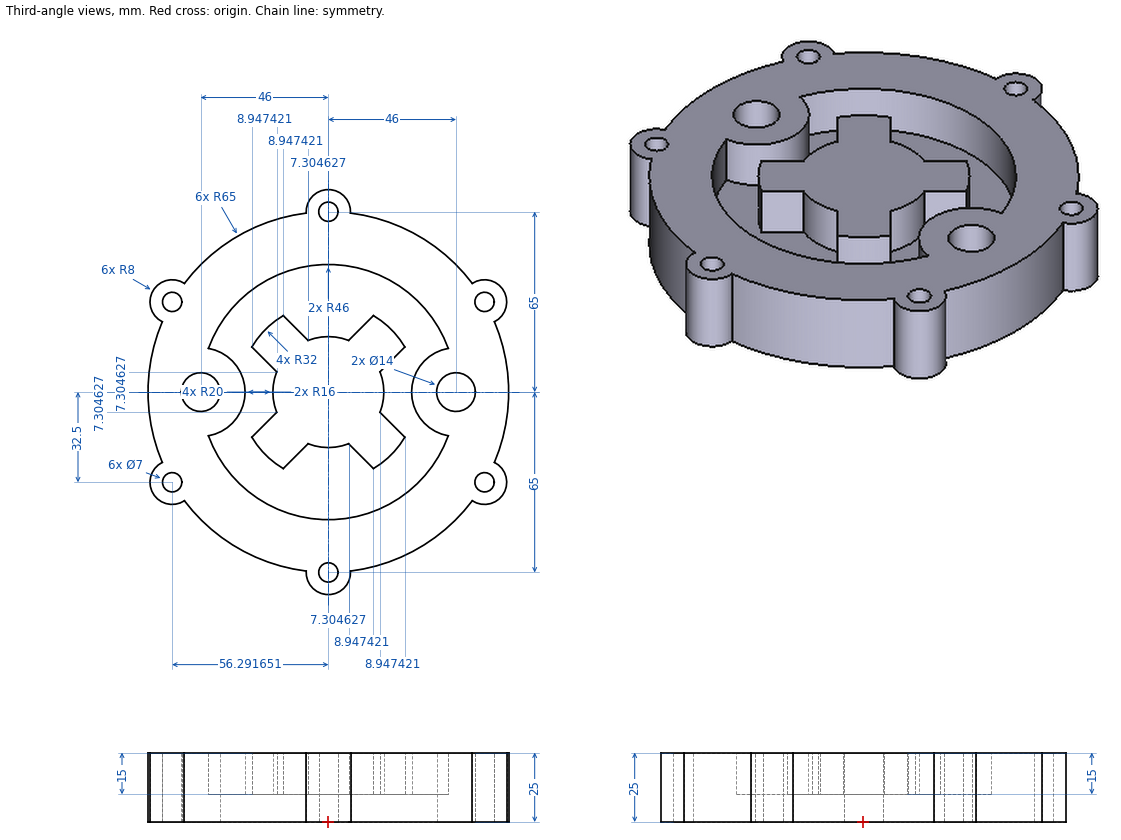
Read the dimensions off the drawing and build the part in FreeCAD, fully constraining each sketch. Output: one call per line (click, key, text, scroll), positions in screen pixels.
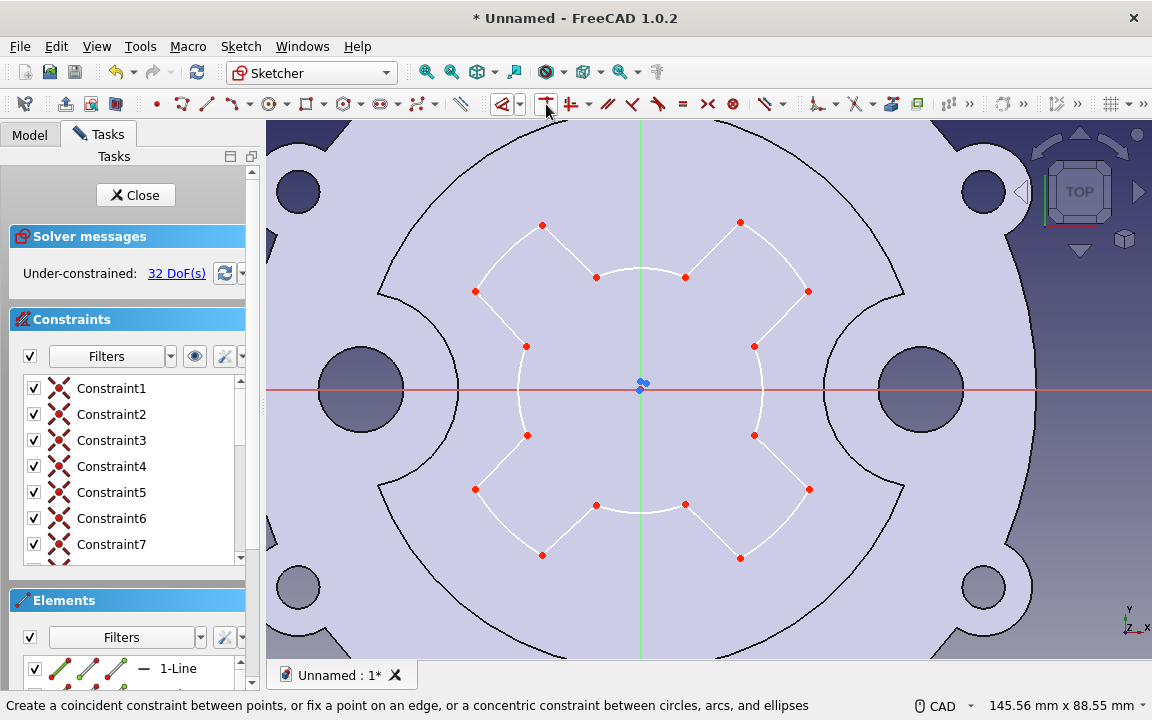
click(519, 241)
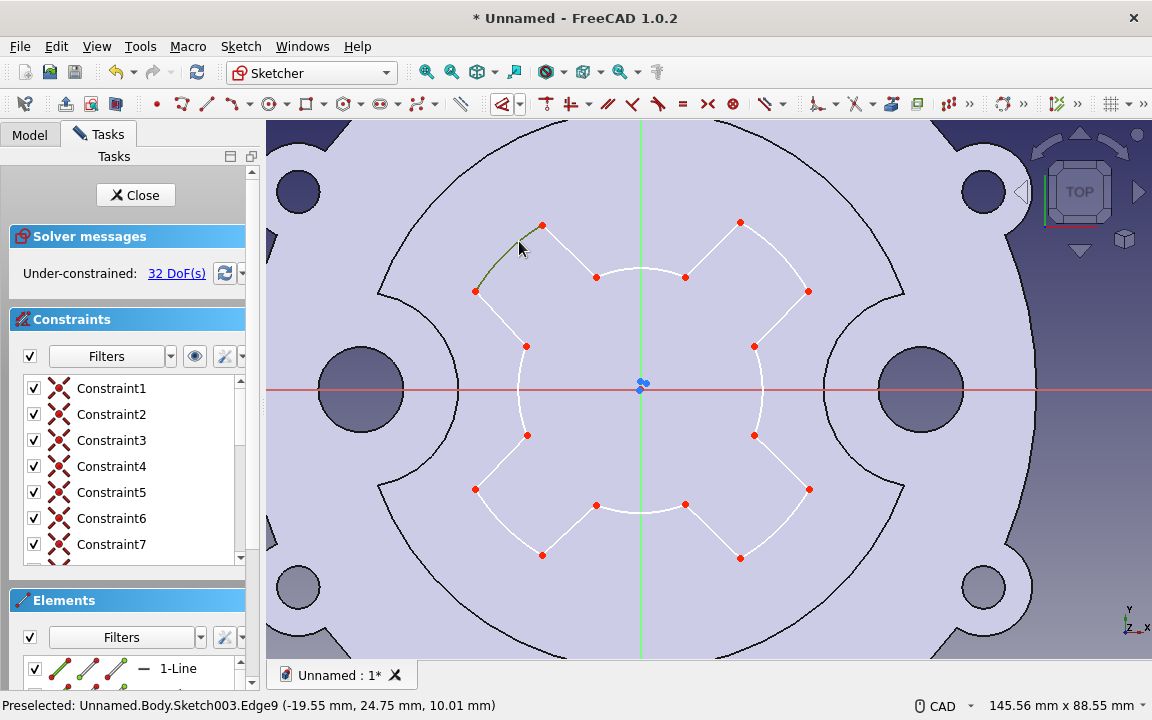
click(761, 409)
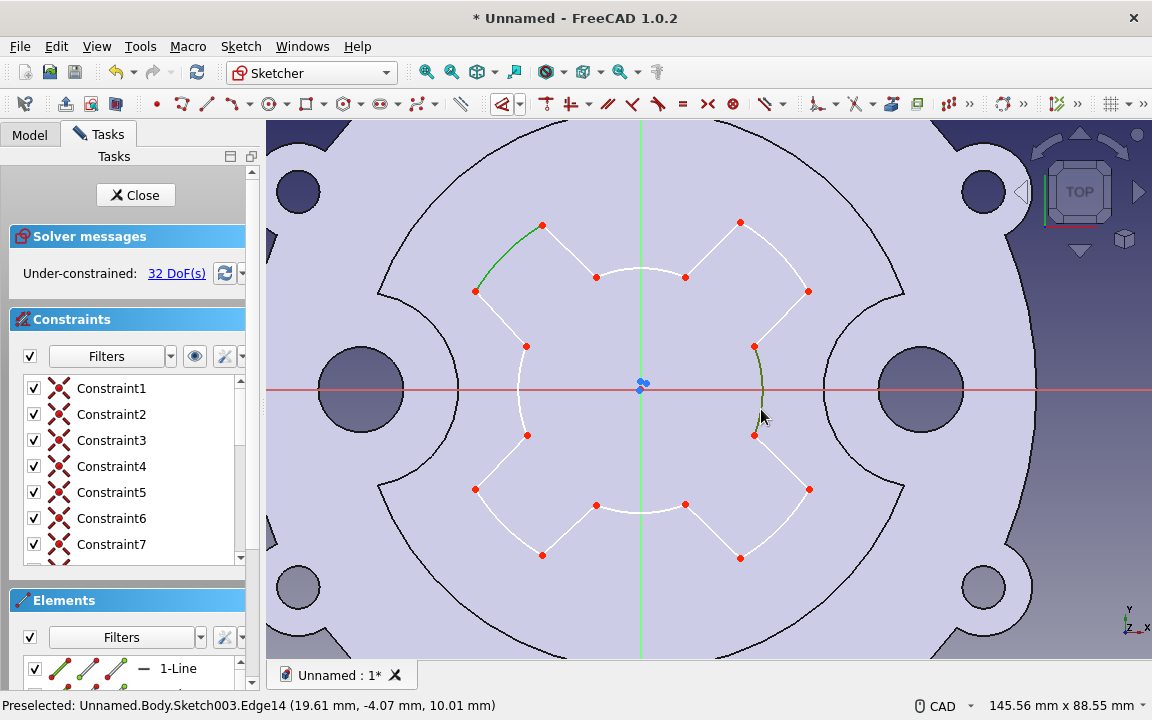
click(546, 104)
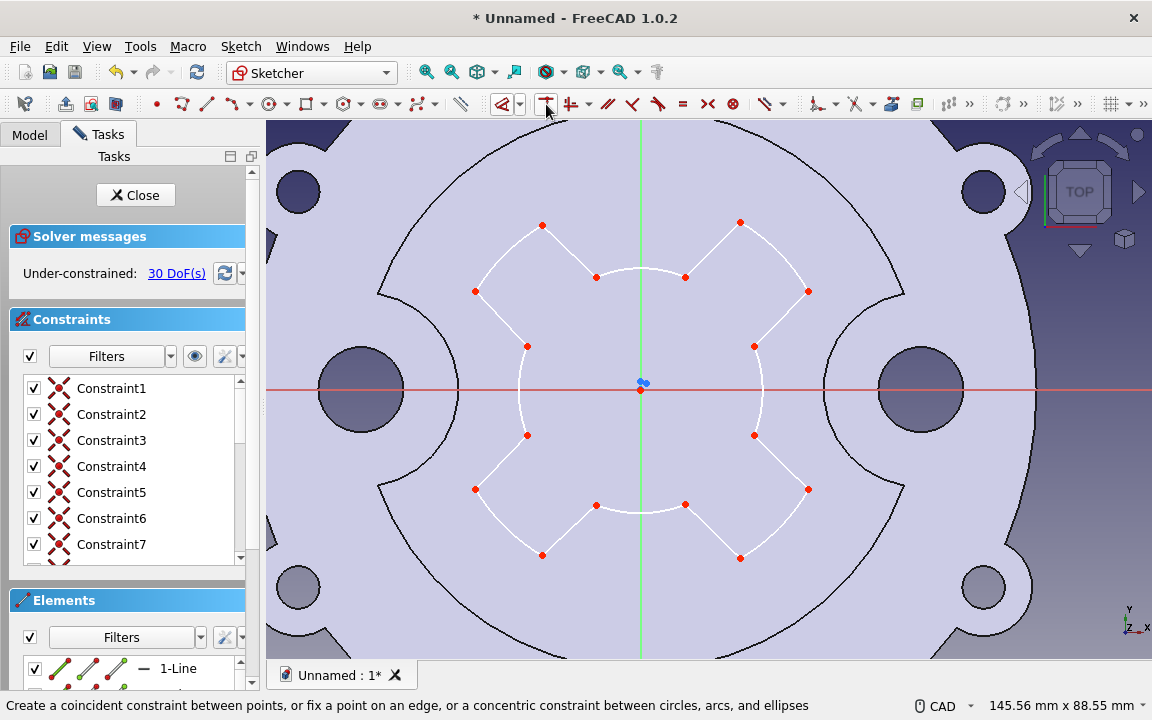
click(519, 242)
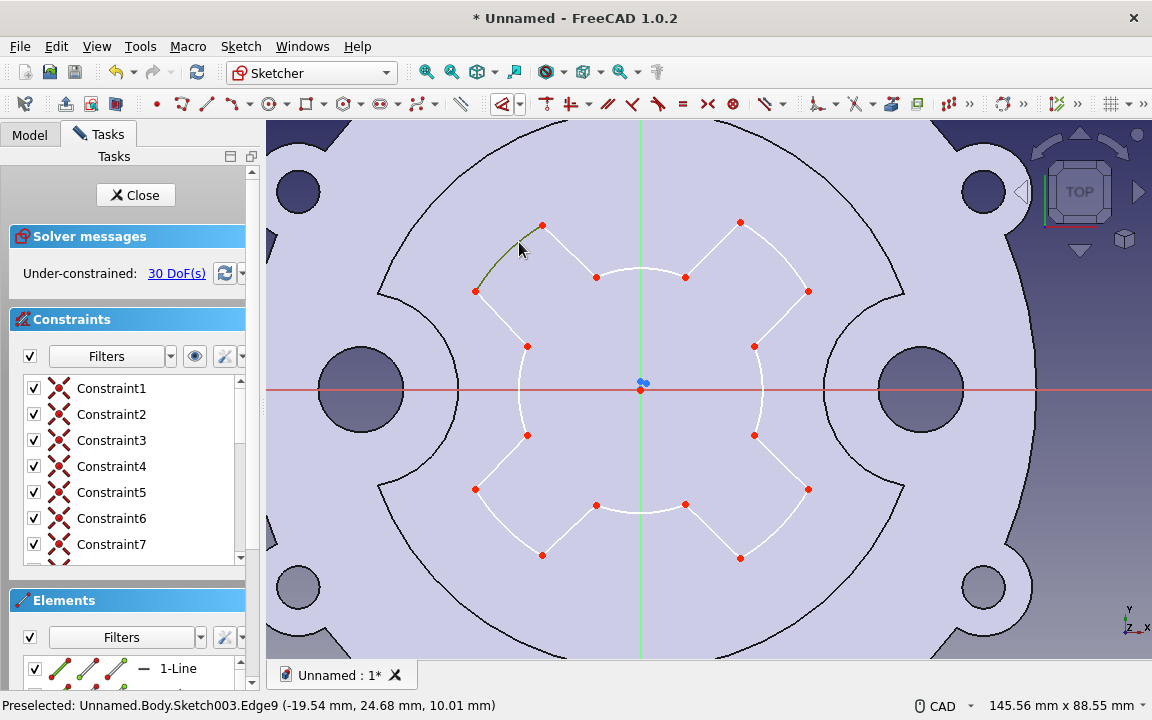
click(792, 267)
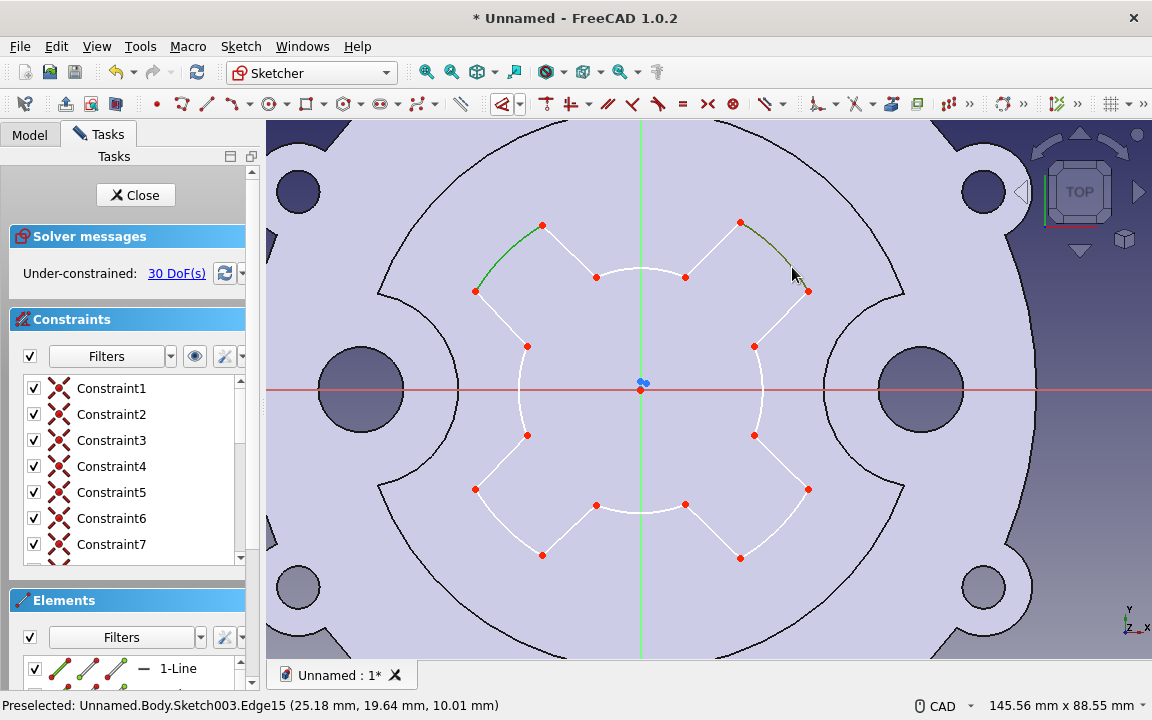
click(546, 104)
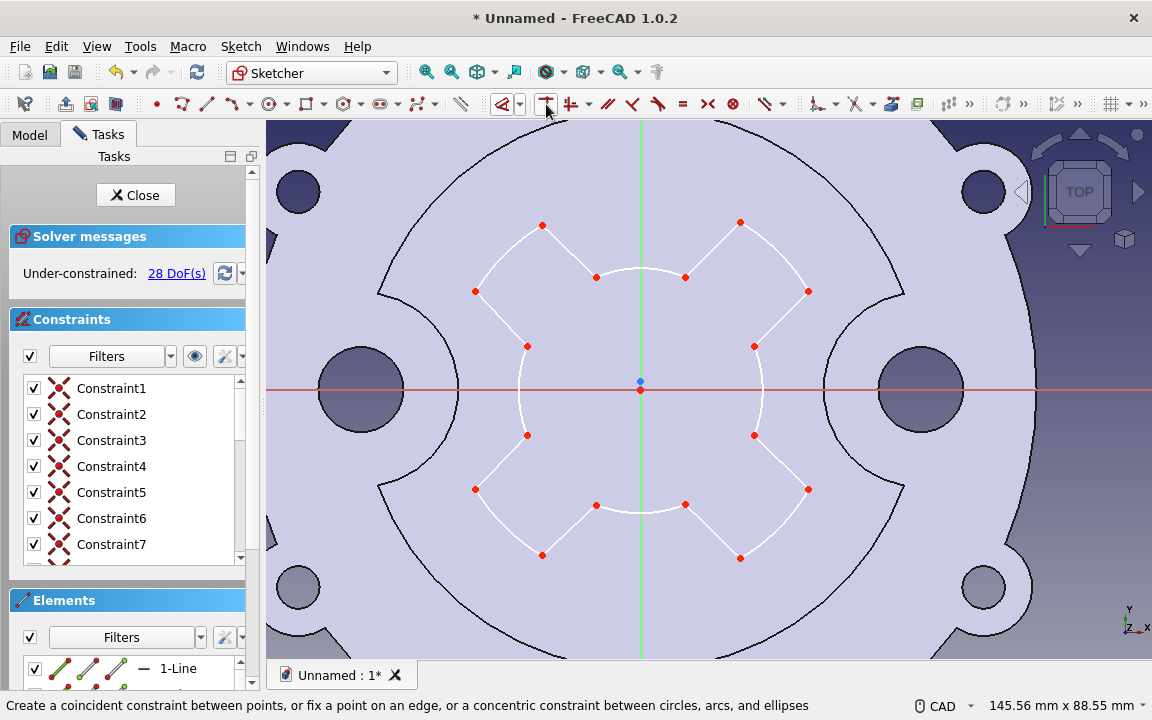
click(519, 242)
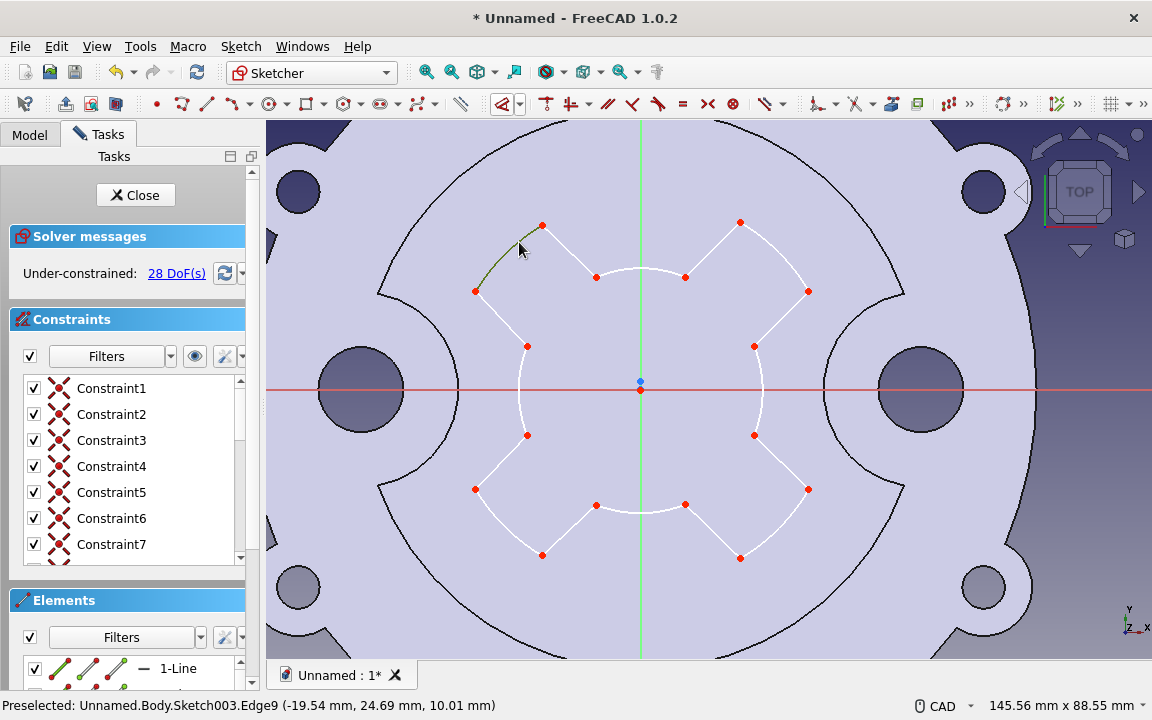
click(659, 270)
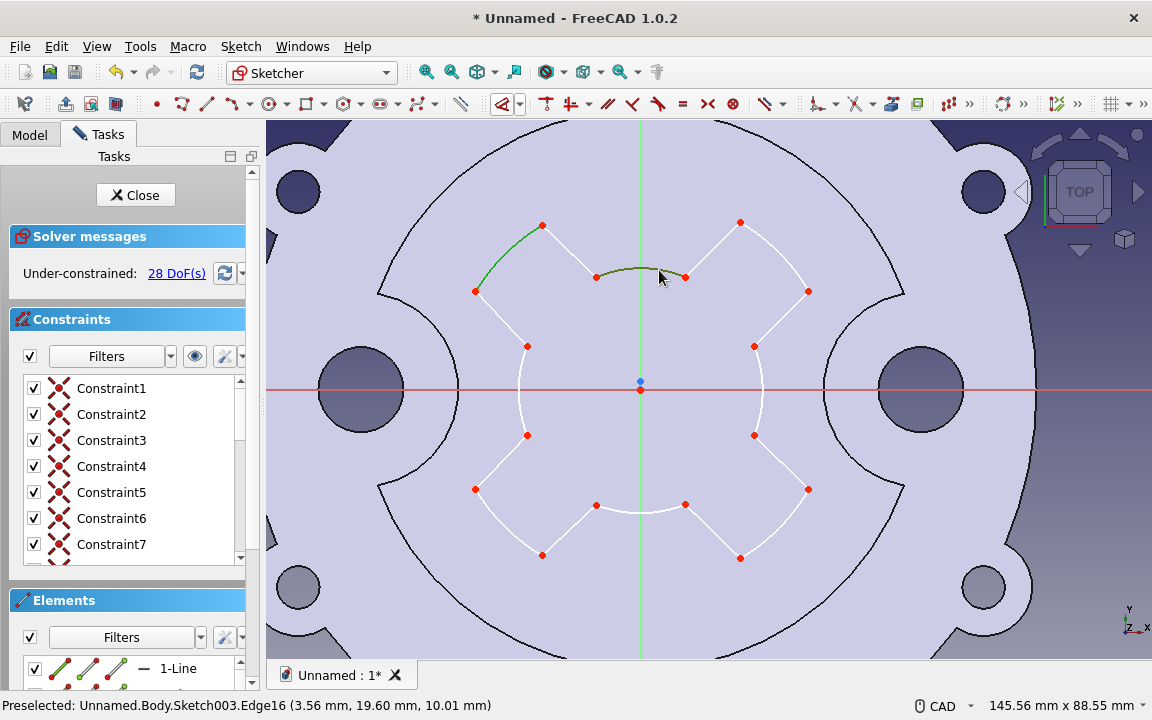
click(546, 104)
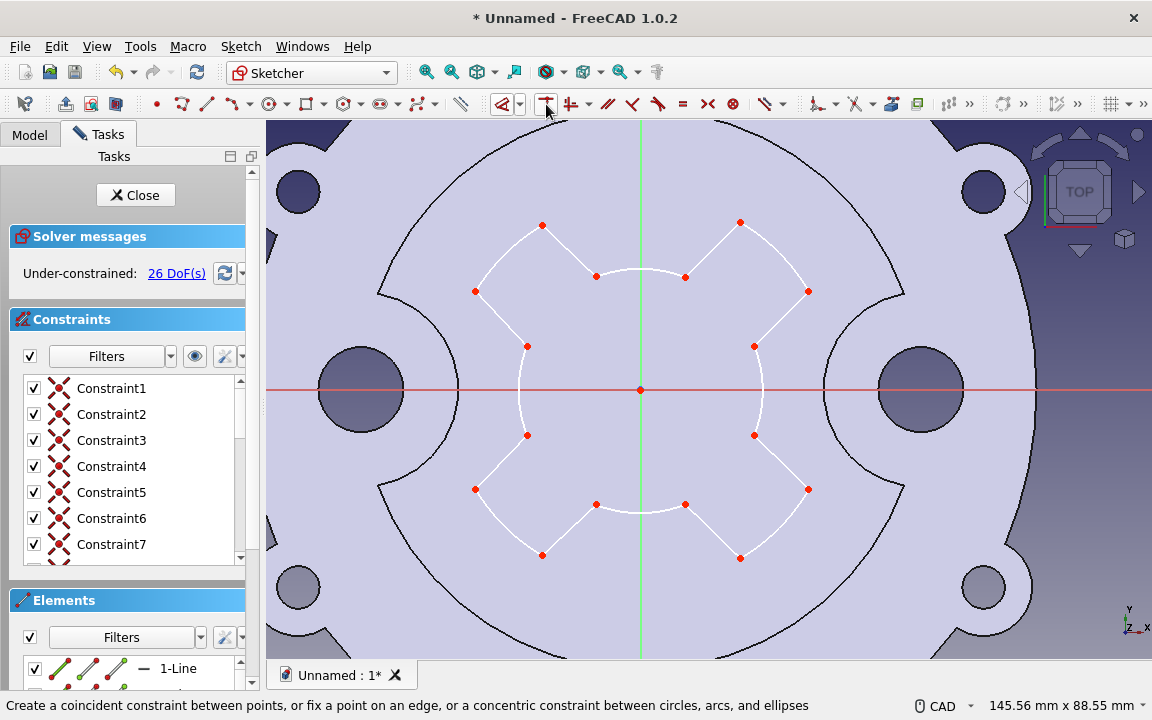
drag(630, 380, 651, 401)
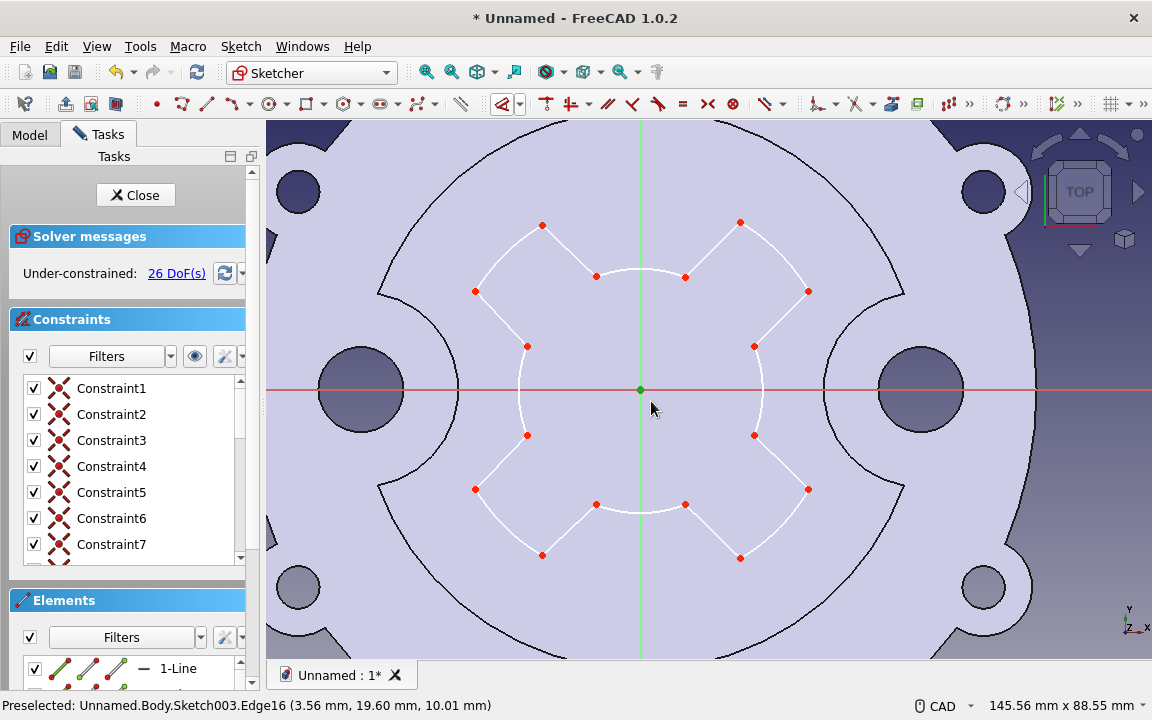
click(546, 104)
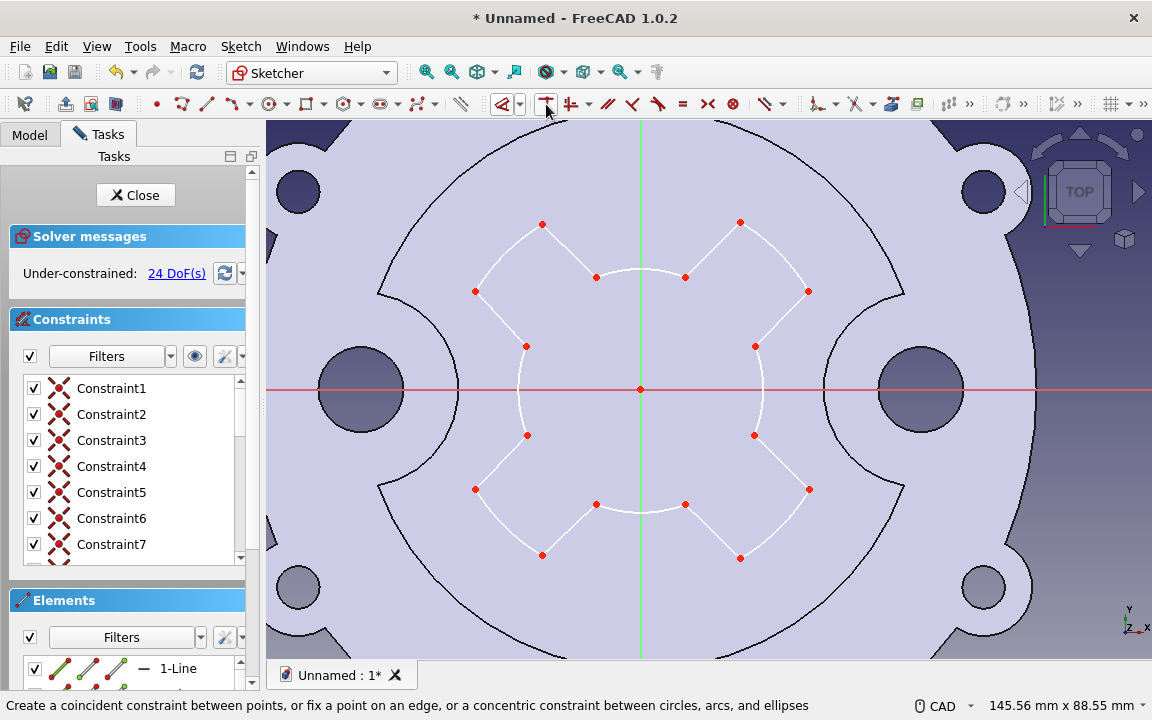
click(519, 241)